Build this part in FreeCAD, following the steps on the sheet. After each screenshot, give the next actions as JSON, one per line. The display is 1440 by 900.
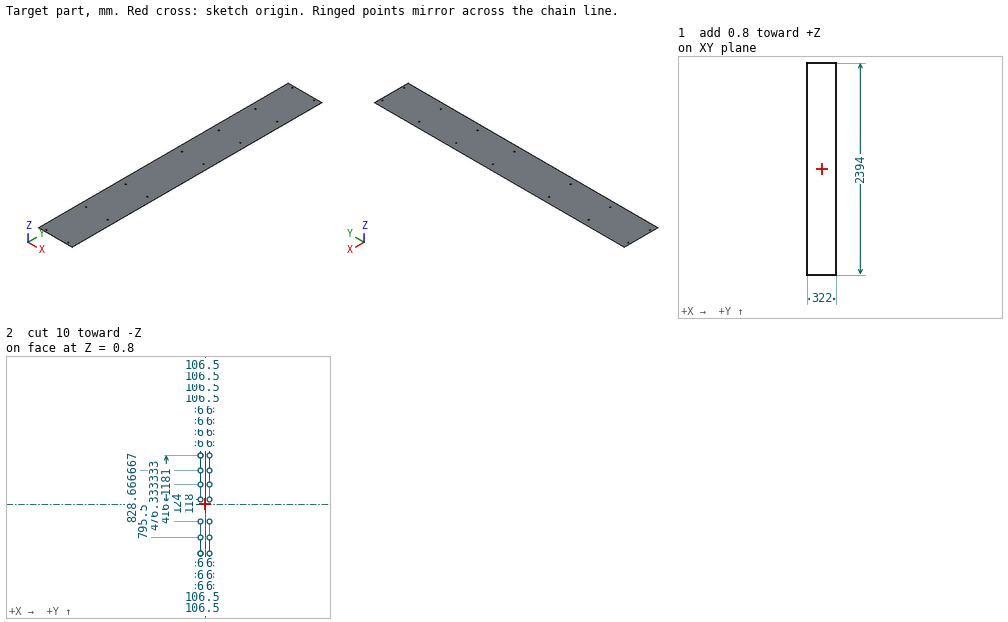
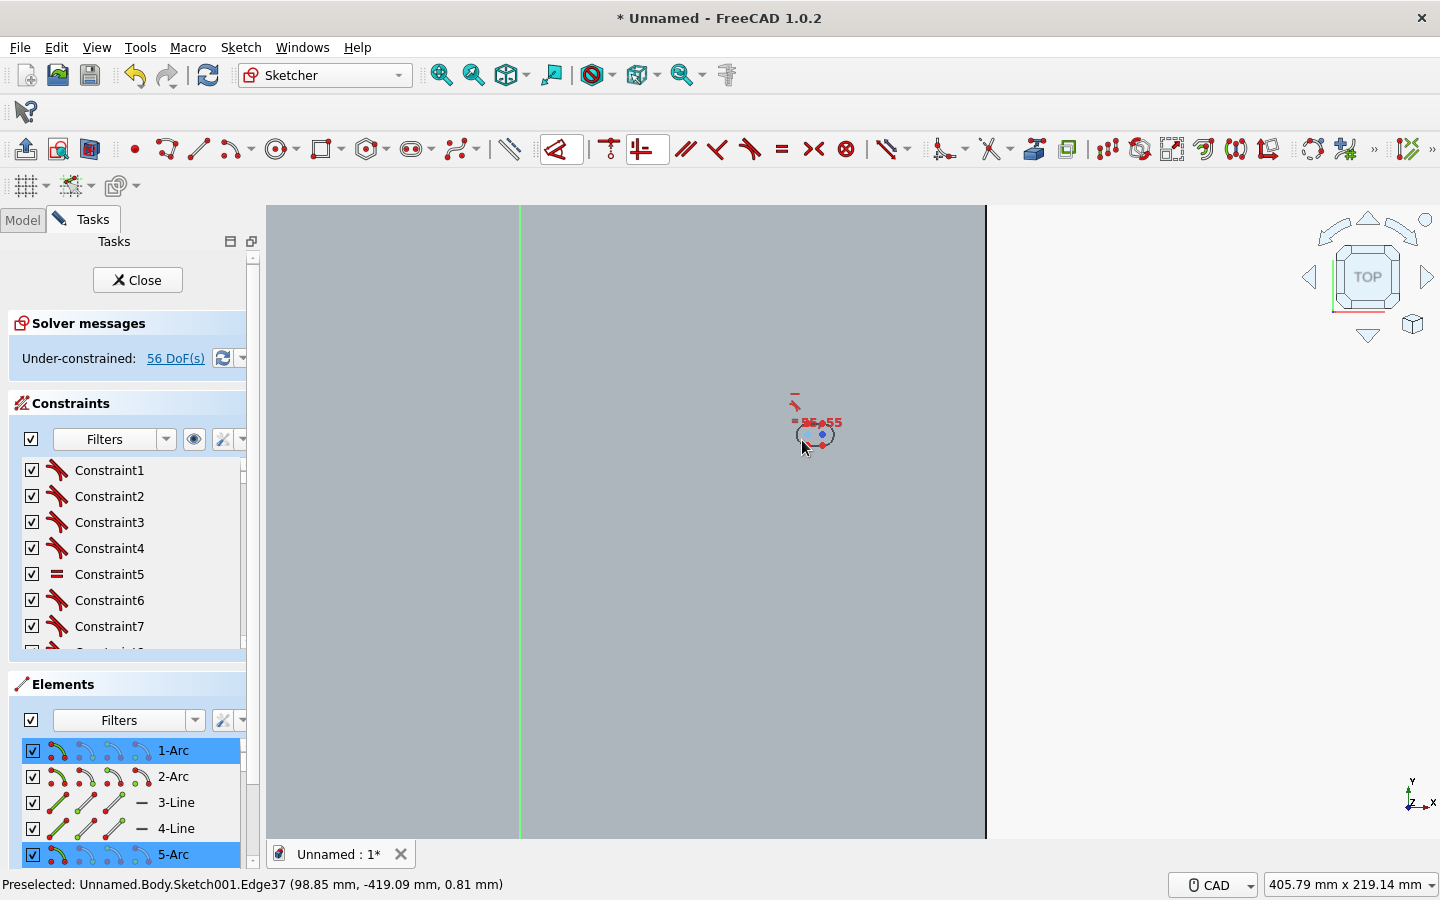
{"action": "left_click", "coordinate": [799, 428]}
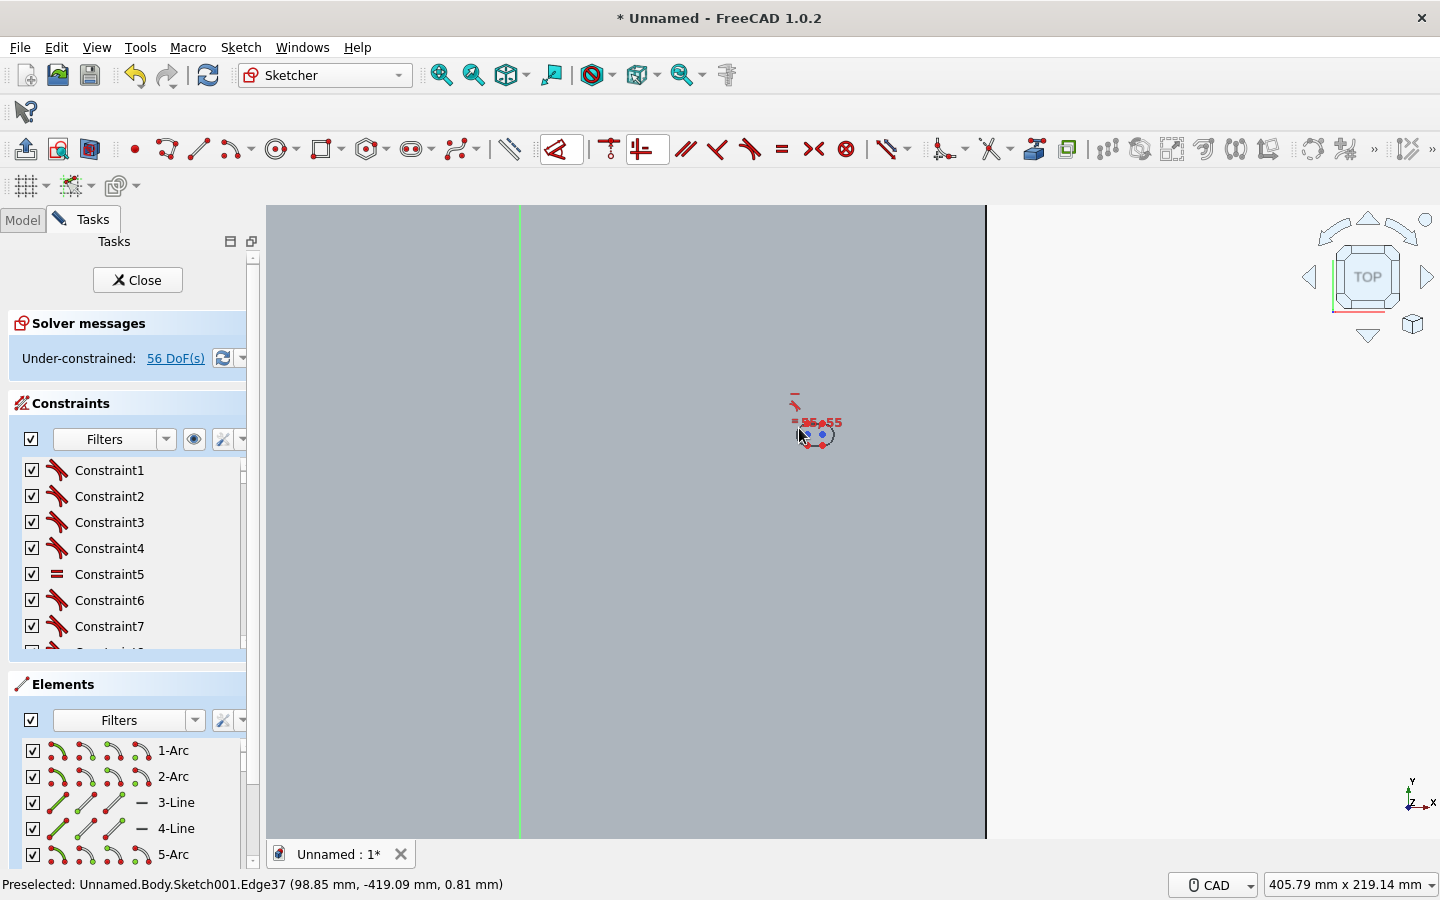
{"action": "scroll", "coordinate": [802, 439], "scroll_direction": "down", "scroll_amount": 14}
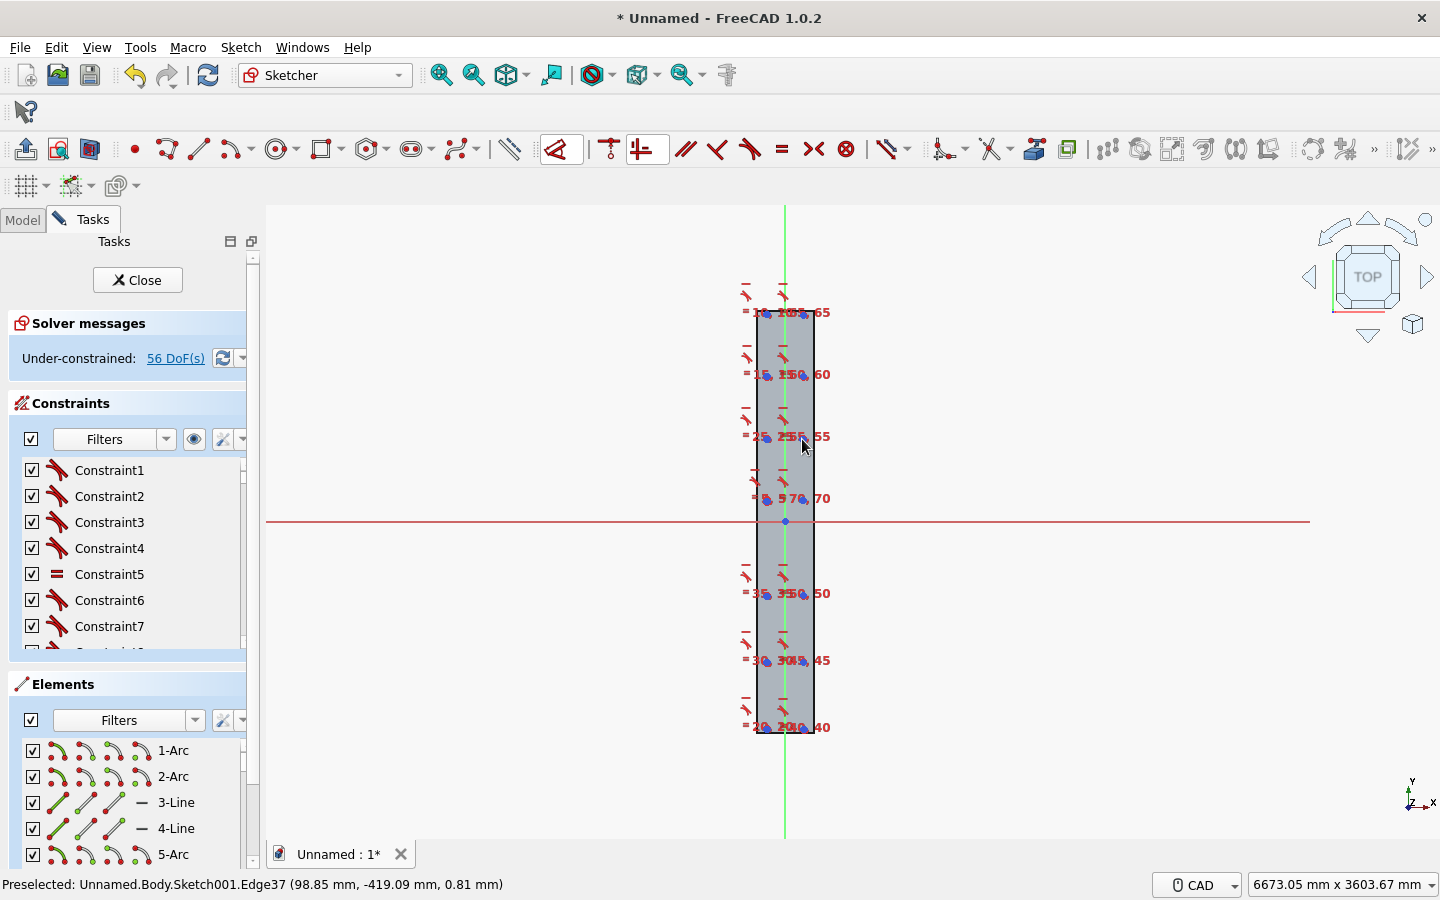
{"action": "scroll", "coordinate": [803, 377], "scroll_direction": "up", "scroll_amount": 14}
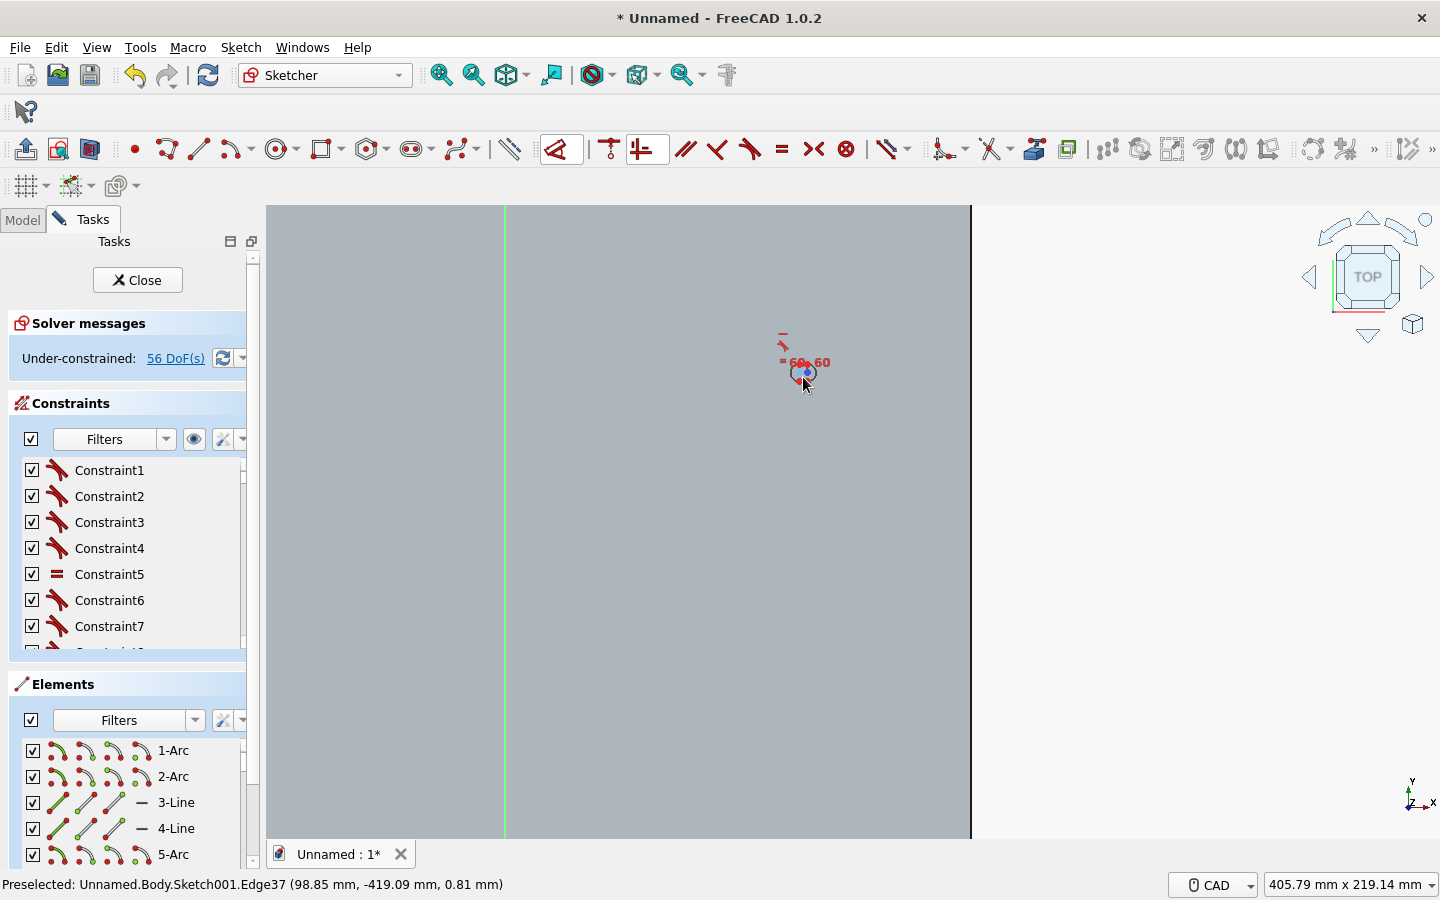
{"action": "left_click", "coordinate": [791, 373]}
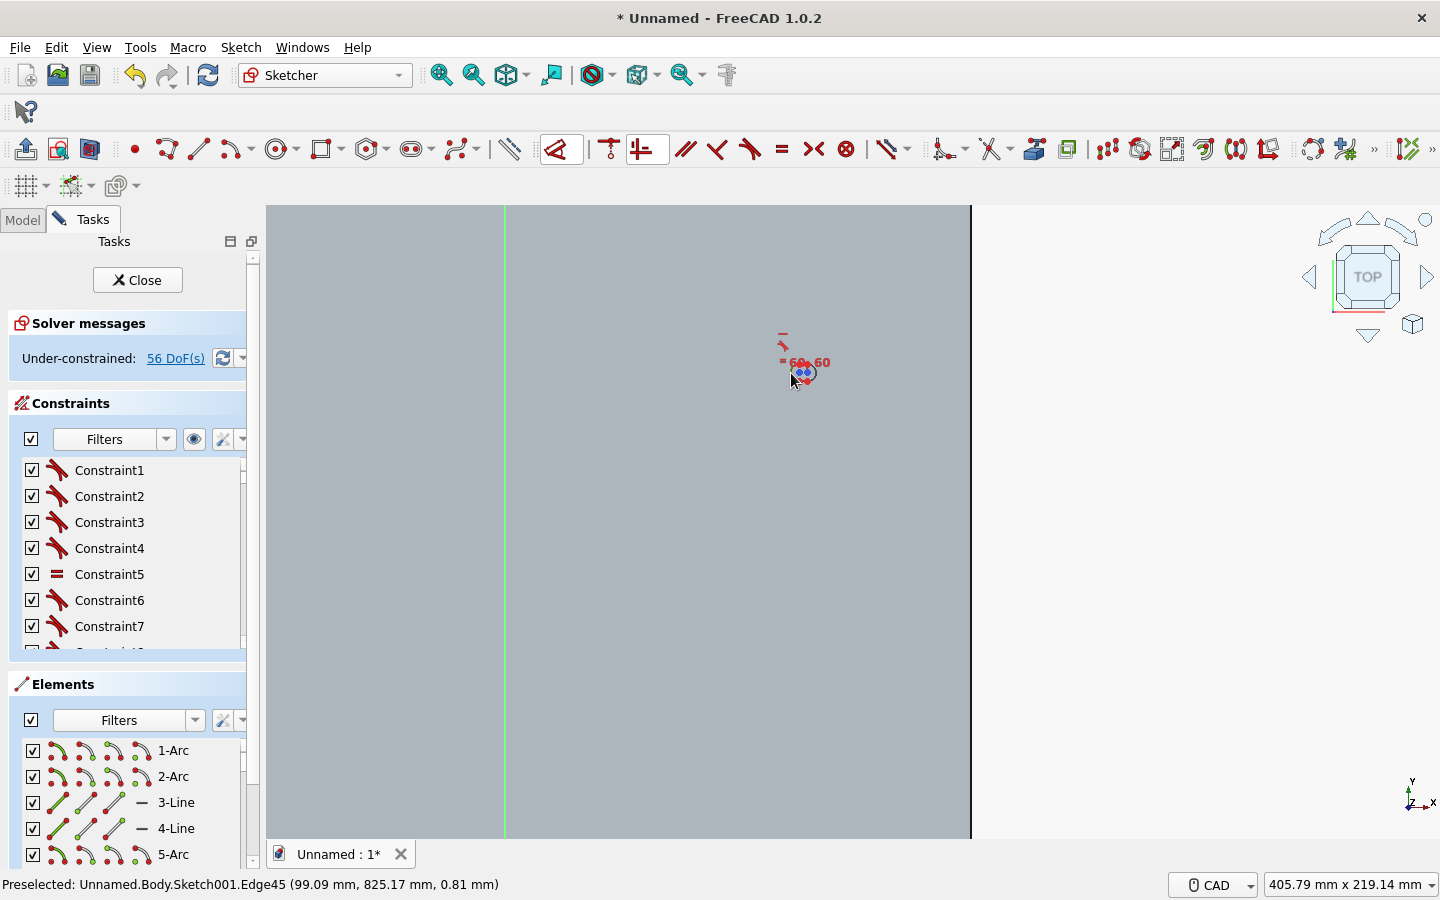
{"action": "scroll", "coordinate": [803, 377], "scroll_direction": "down", "scroll_amount": 14}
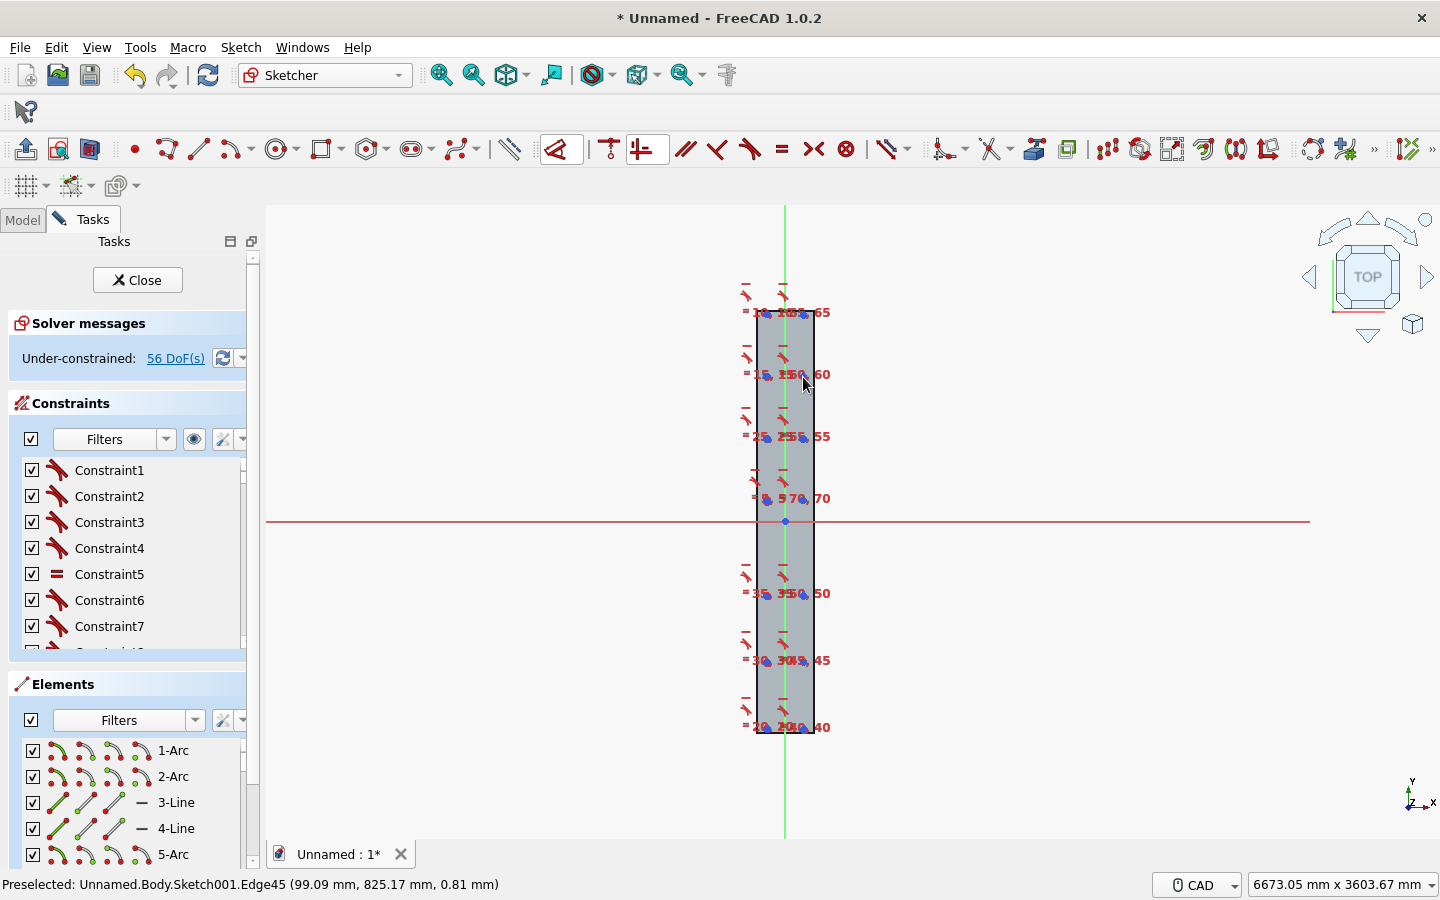
{"action": "scroll", "coordinate": [803, 315], "scroll_direction": "up", "scroll_amount": 14}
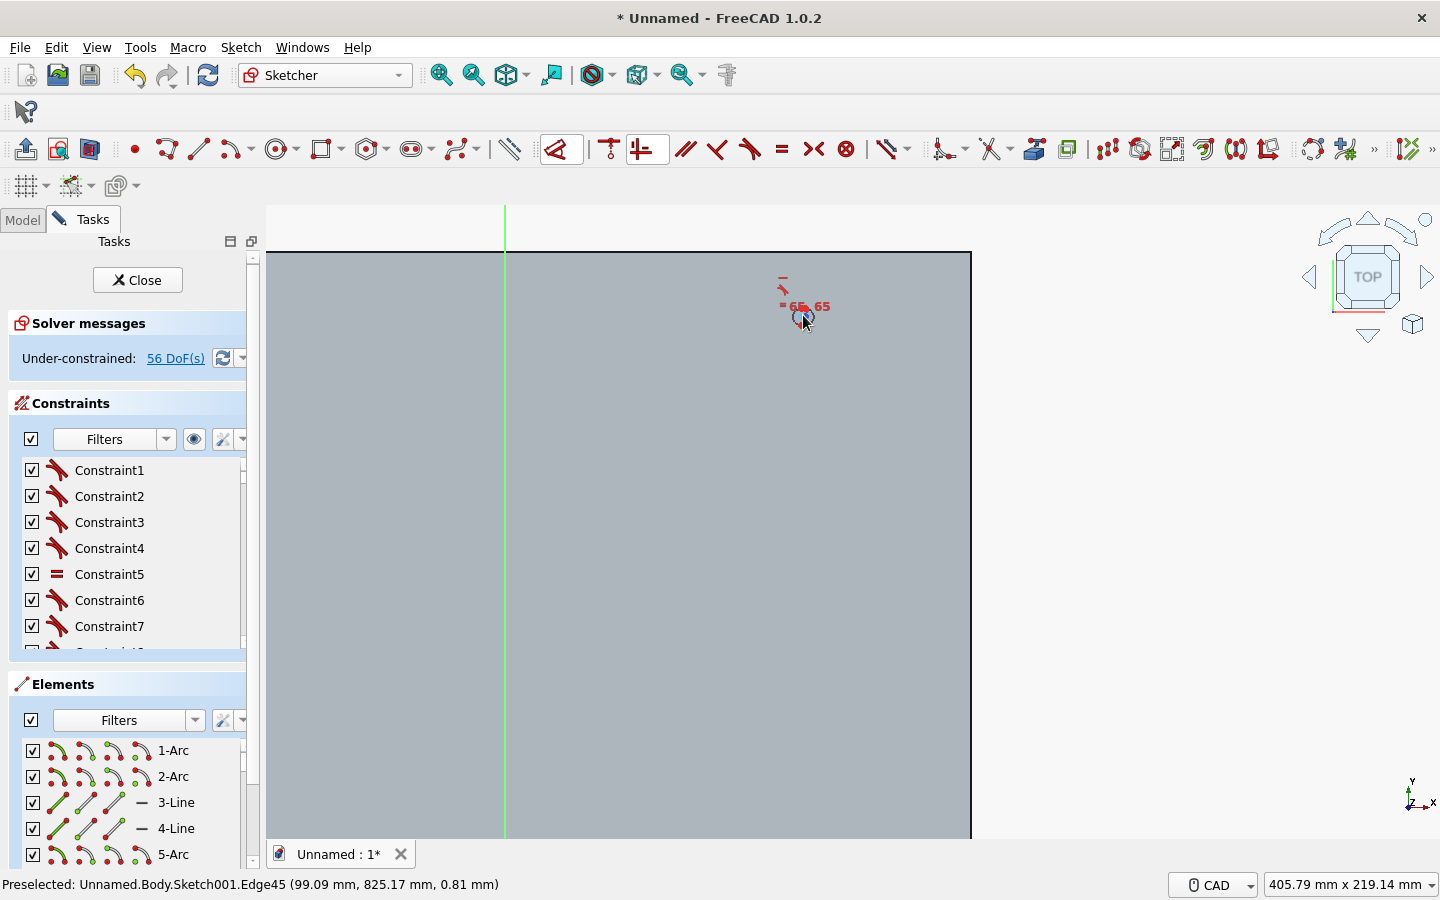
{"action": "left_click", "coordinate": [793, 317]}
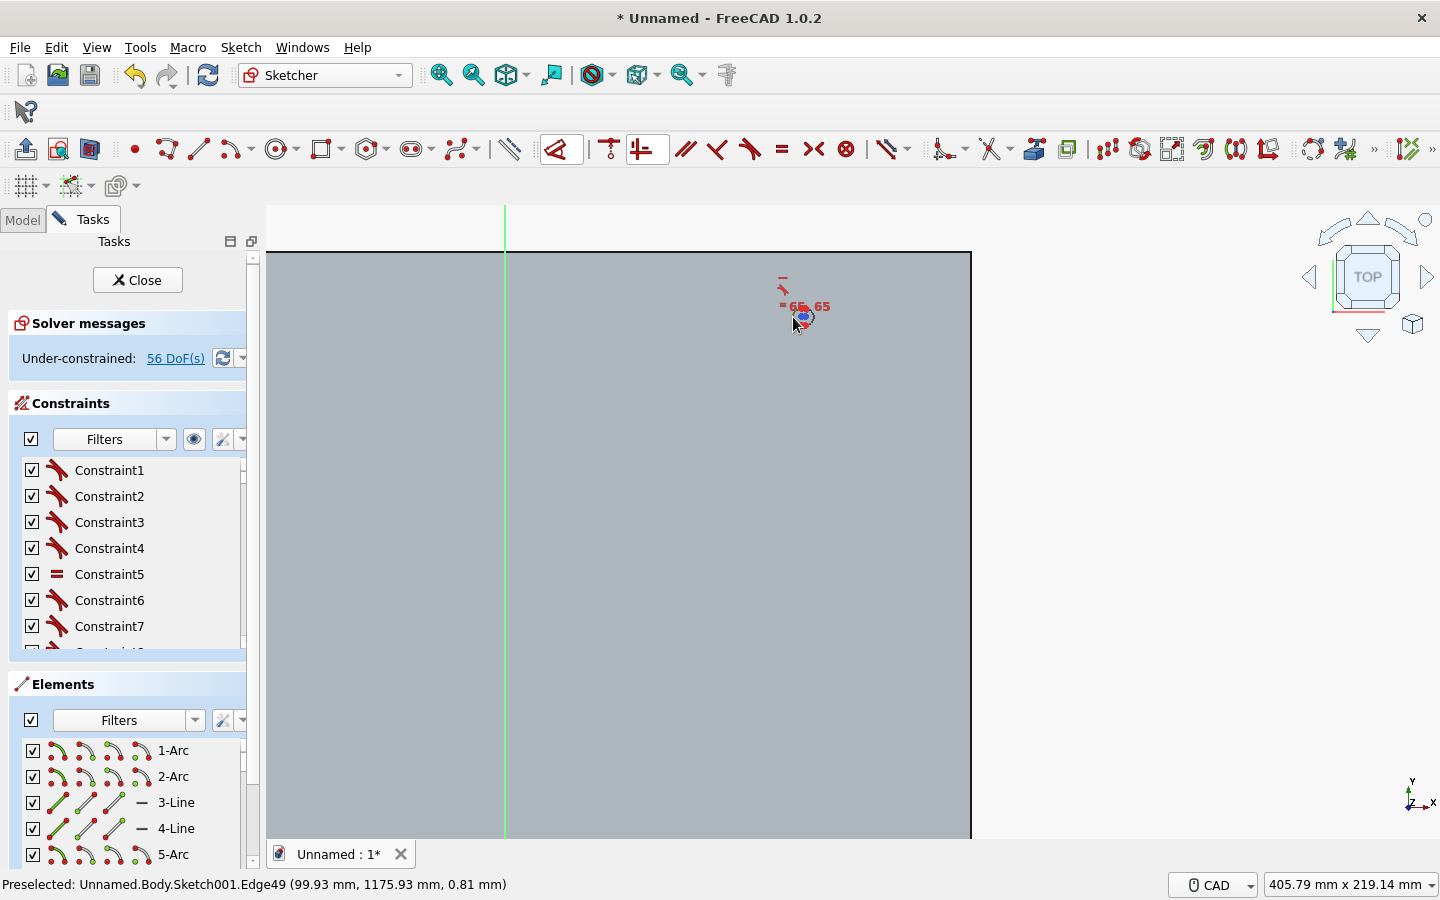
{"action": "scroll", "coordinate": [803, 315], "scroll_direction": "down", "scroll_amount": 14}